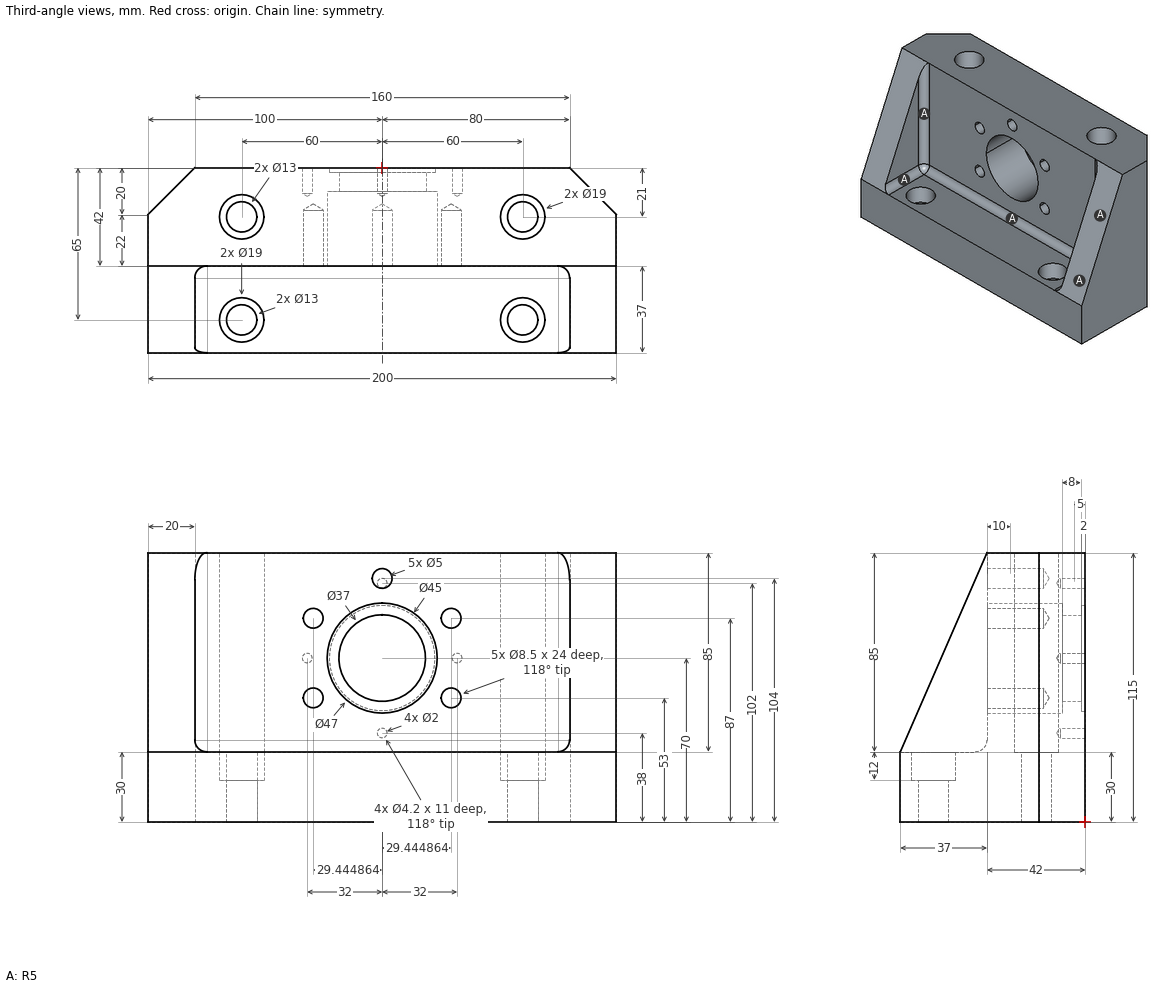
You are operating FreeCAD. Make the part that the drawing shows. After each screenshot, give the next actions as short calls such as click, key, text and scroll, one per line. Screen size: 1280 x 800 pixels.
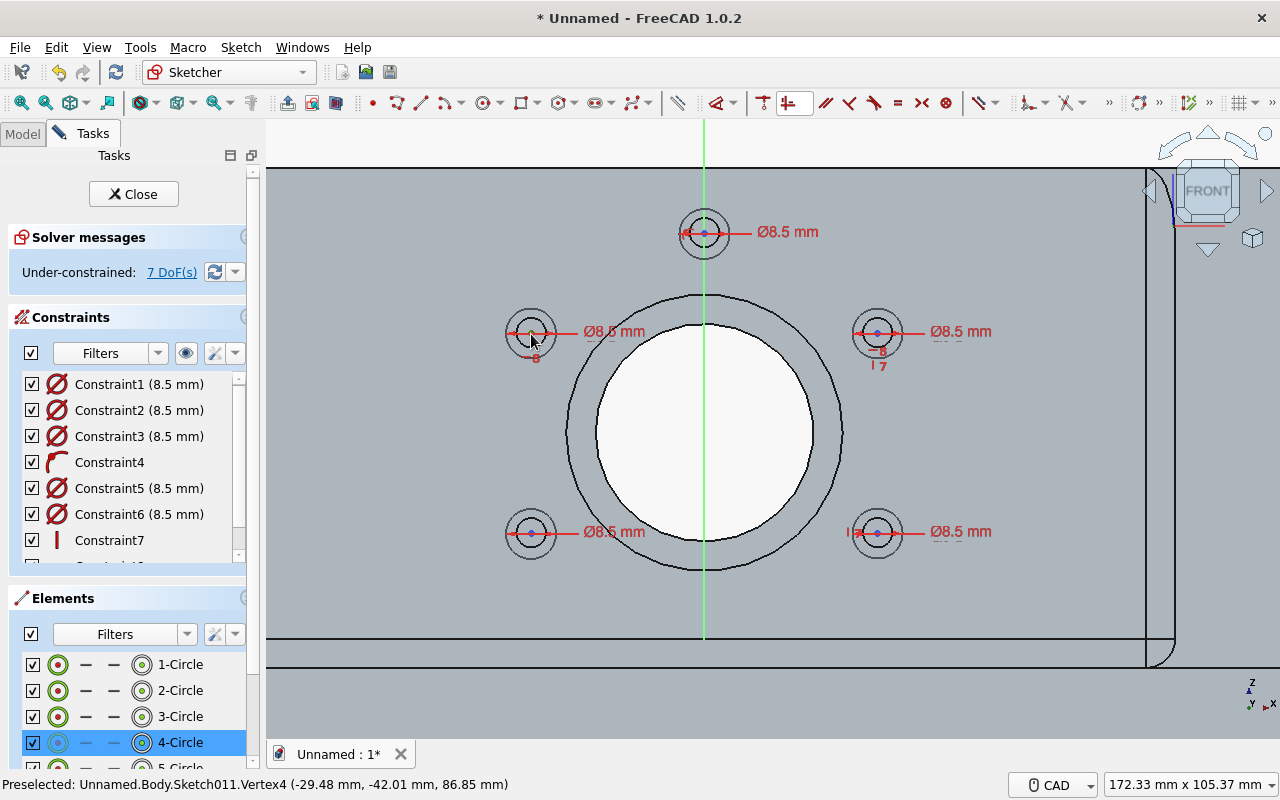
click(531, 534)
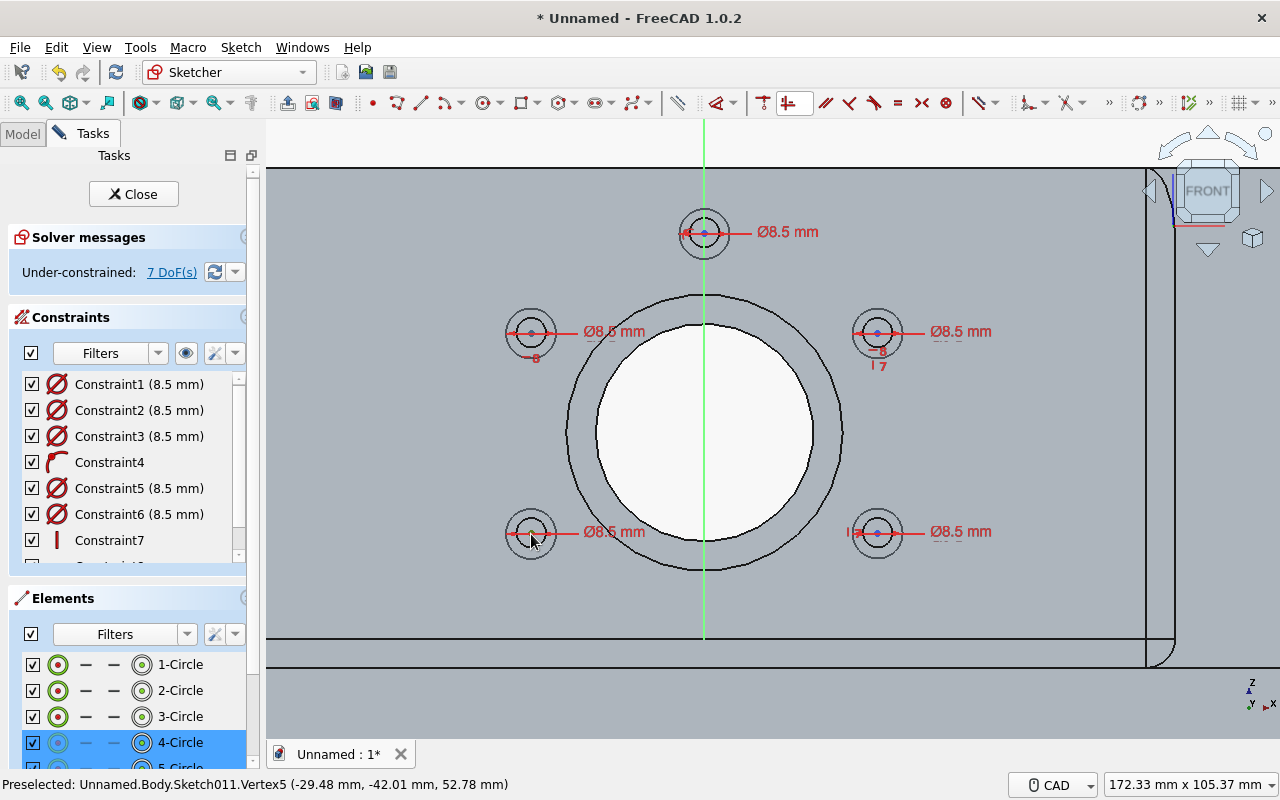
key(v)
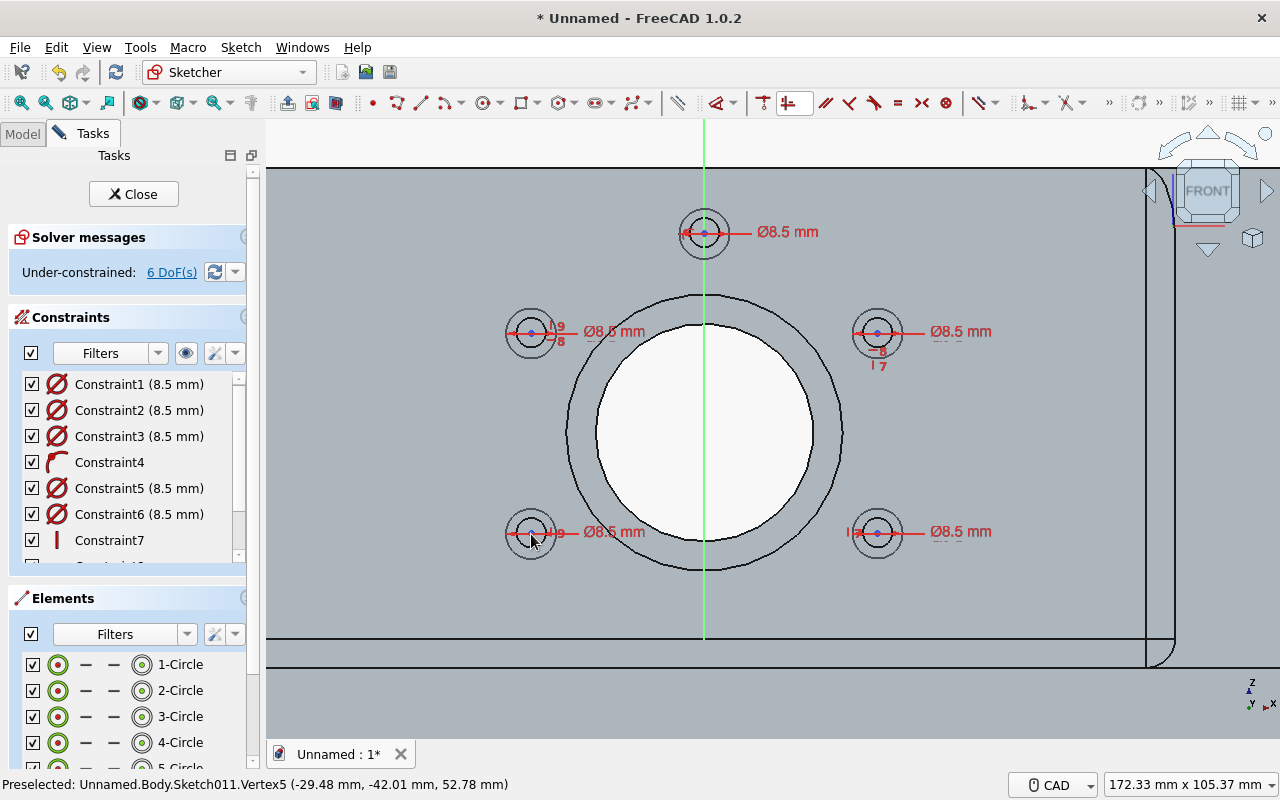
click(878, 534)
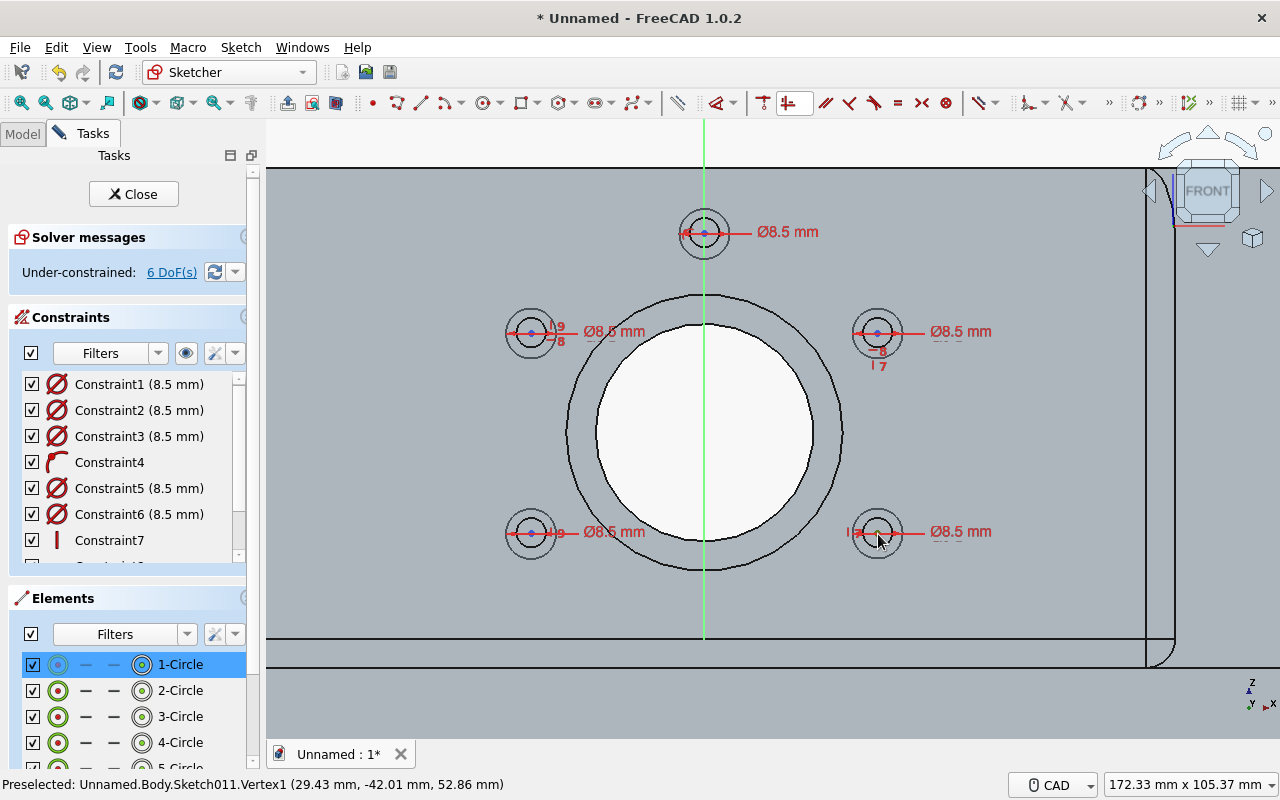
click(531, 534)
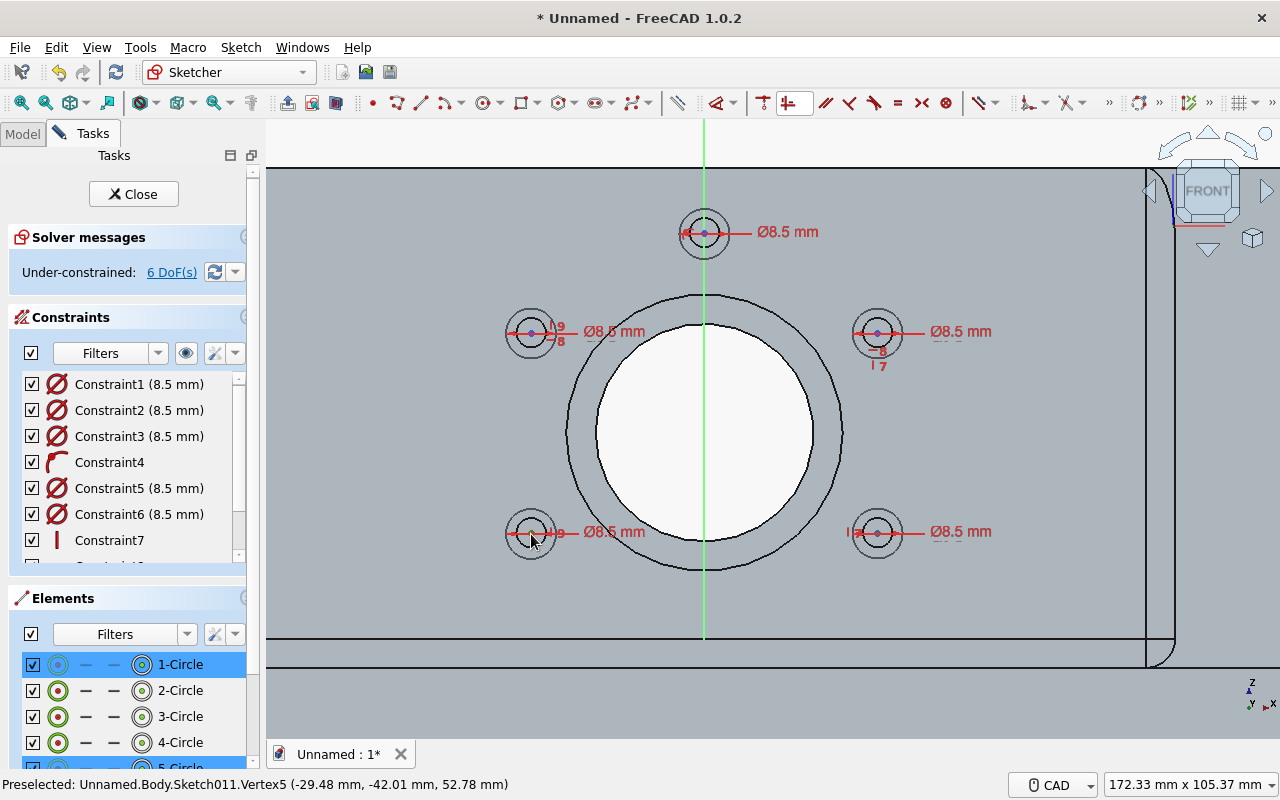
click(808, 104)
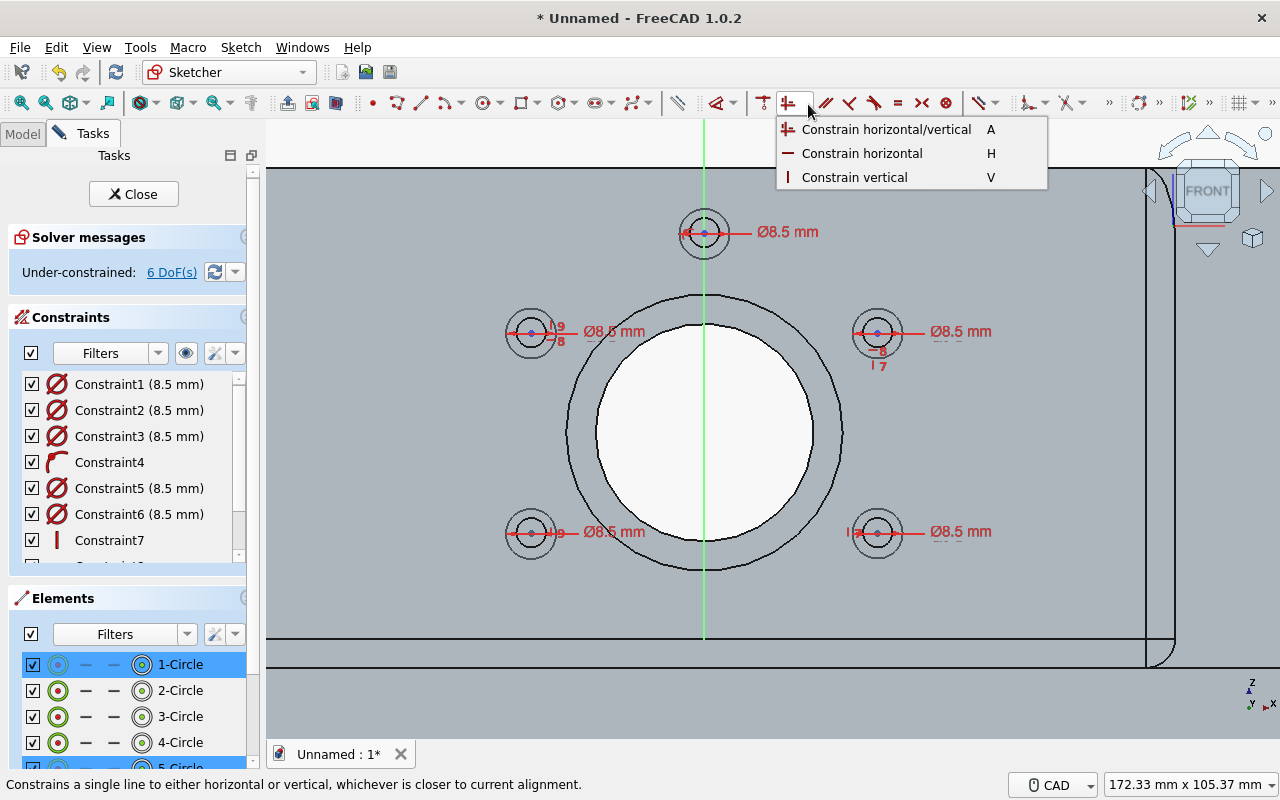
click(912, 153)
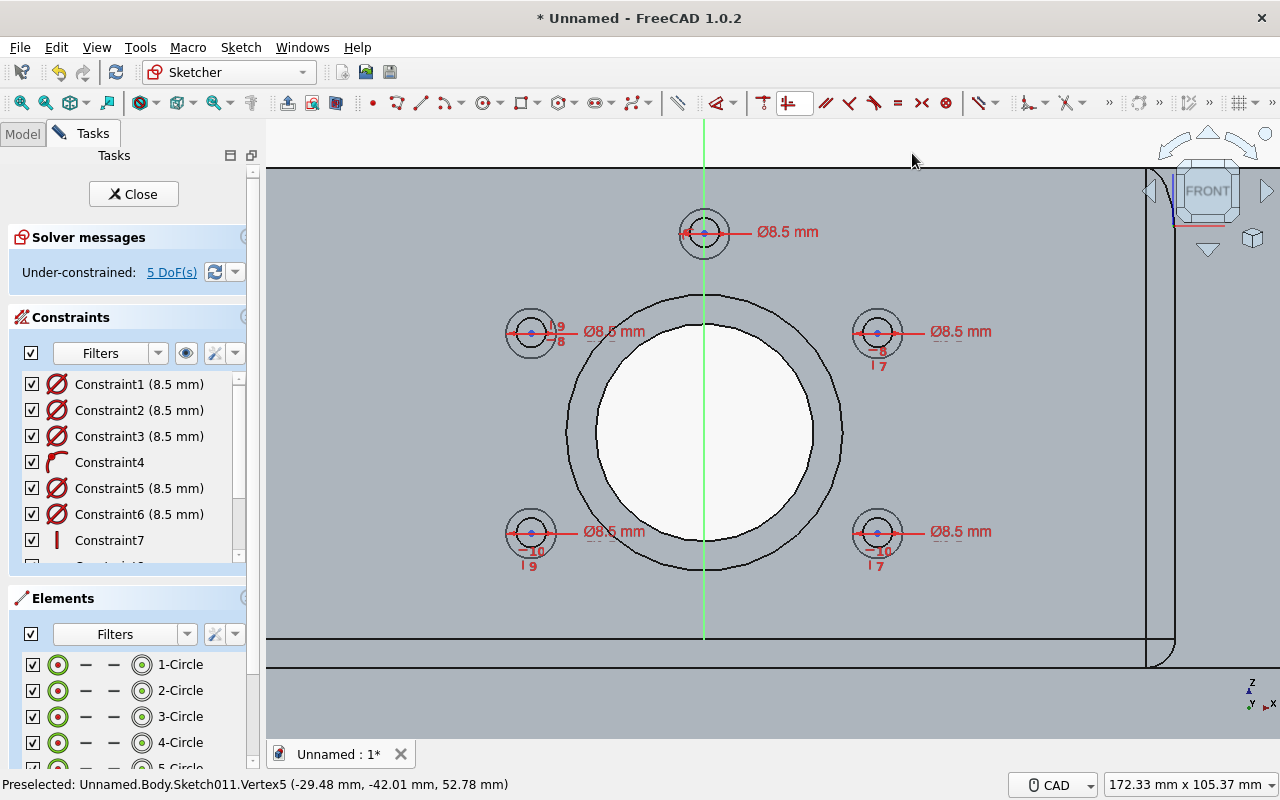
click(716, 104)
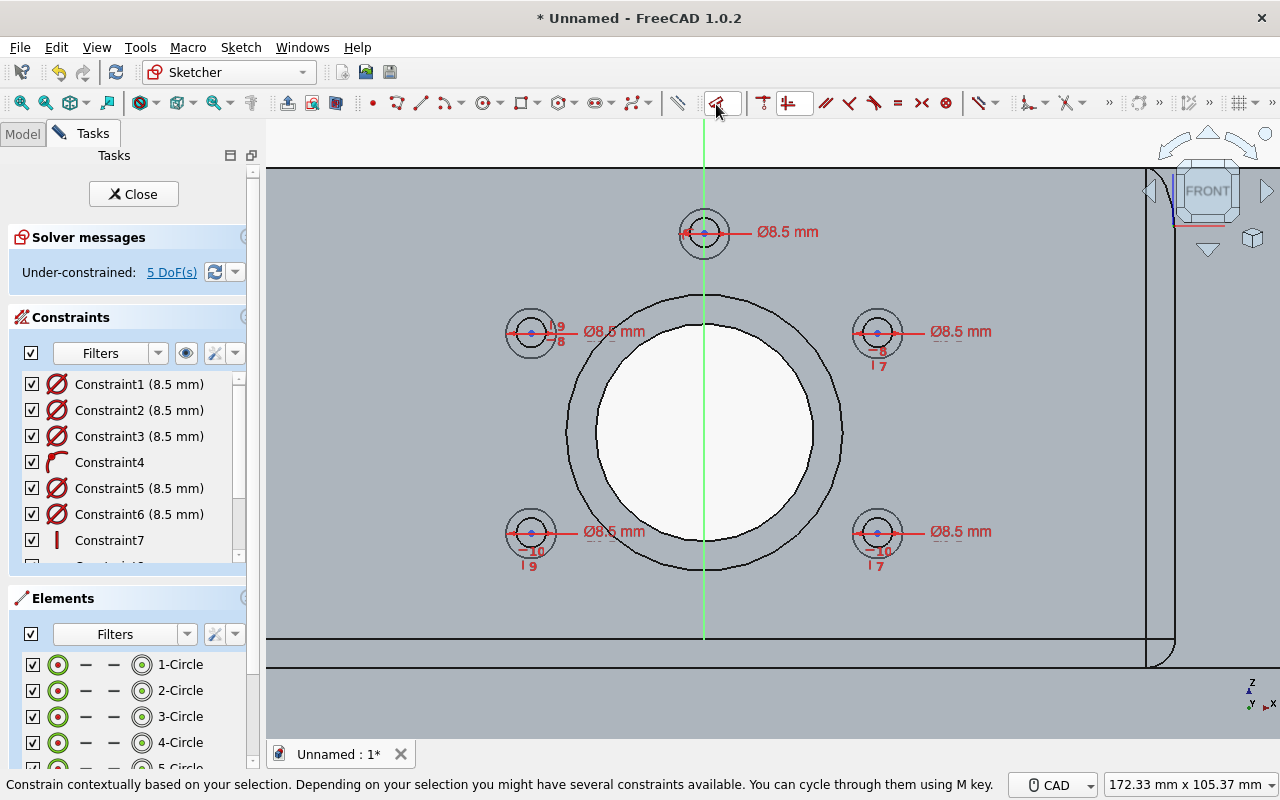
click(878, 534)
click(912, 622)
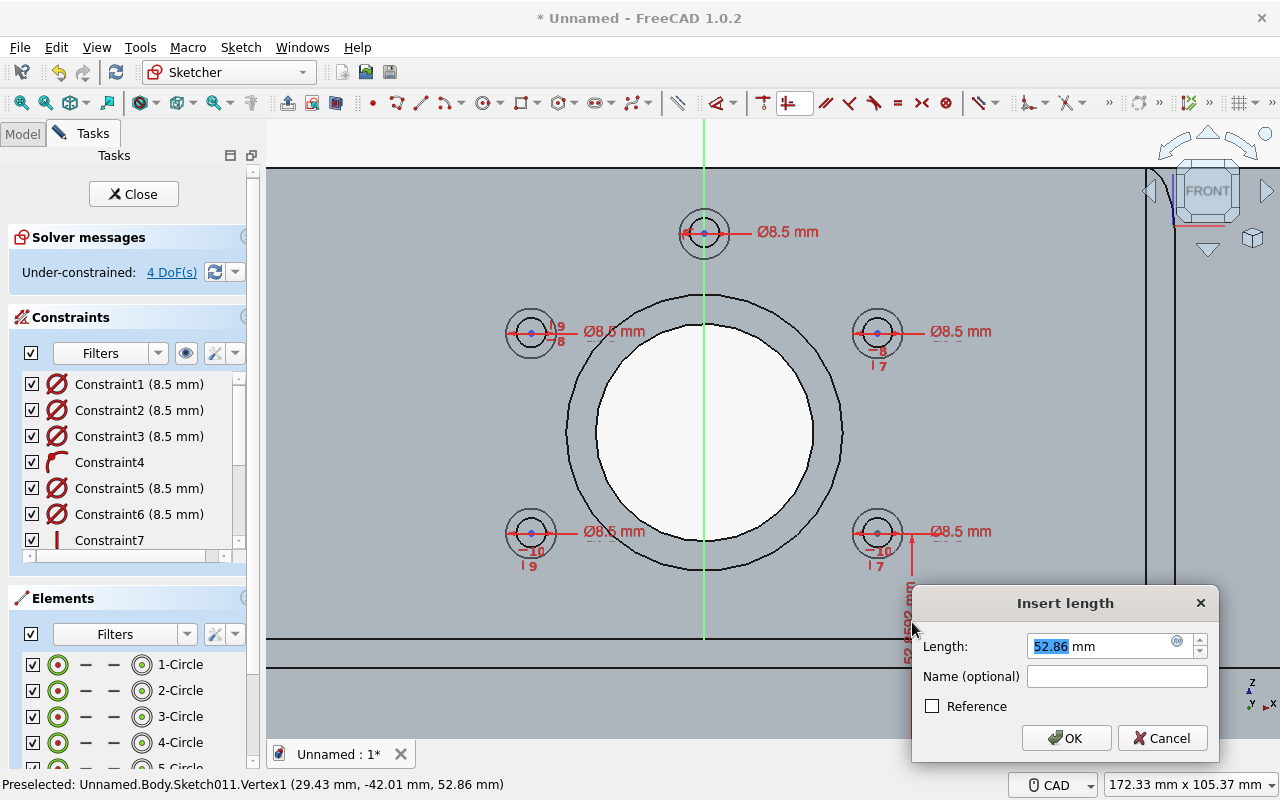
text(53)
key(Return)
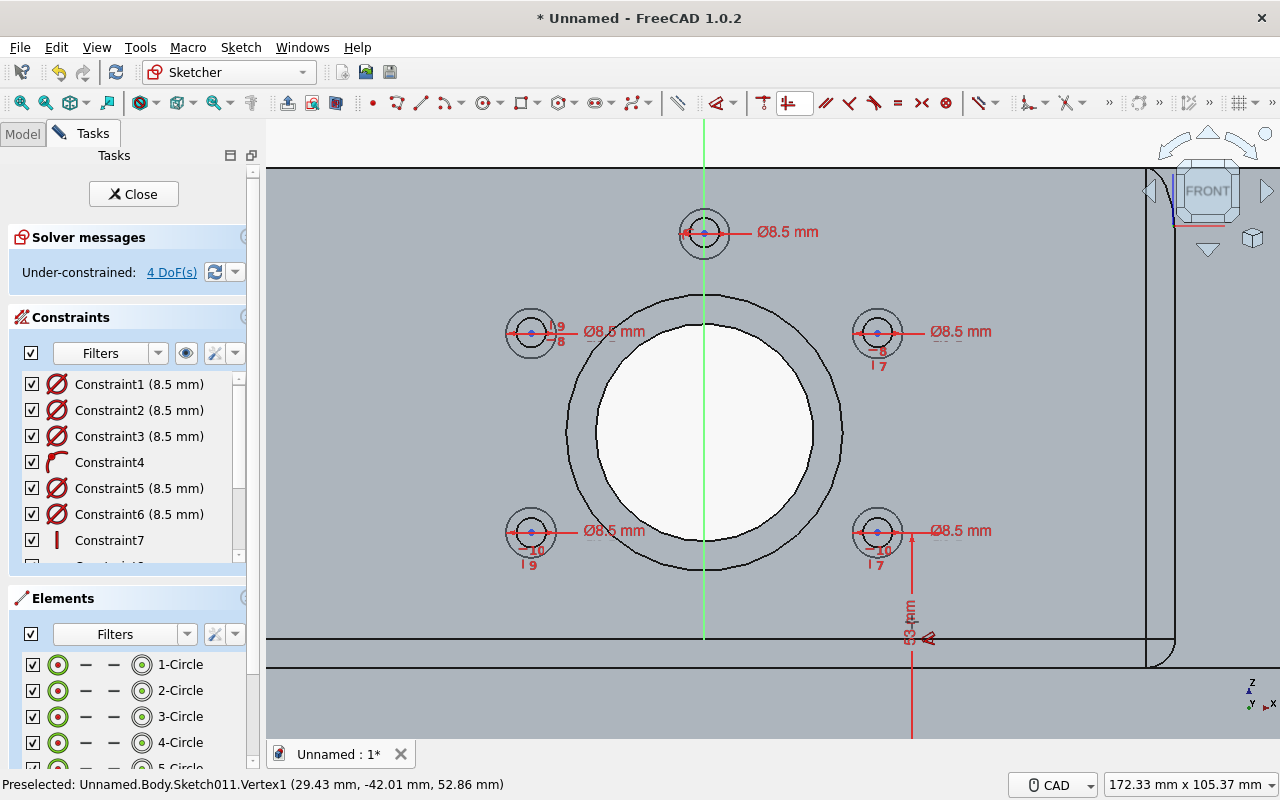
click(878, 334)
click(912, 435)